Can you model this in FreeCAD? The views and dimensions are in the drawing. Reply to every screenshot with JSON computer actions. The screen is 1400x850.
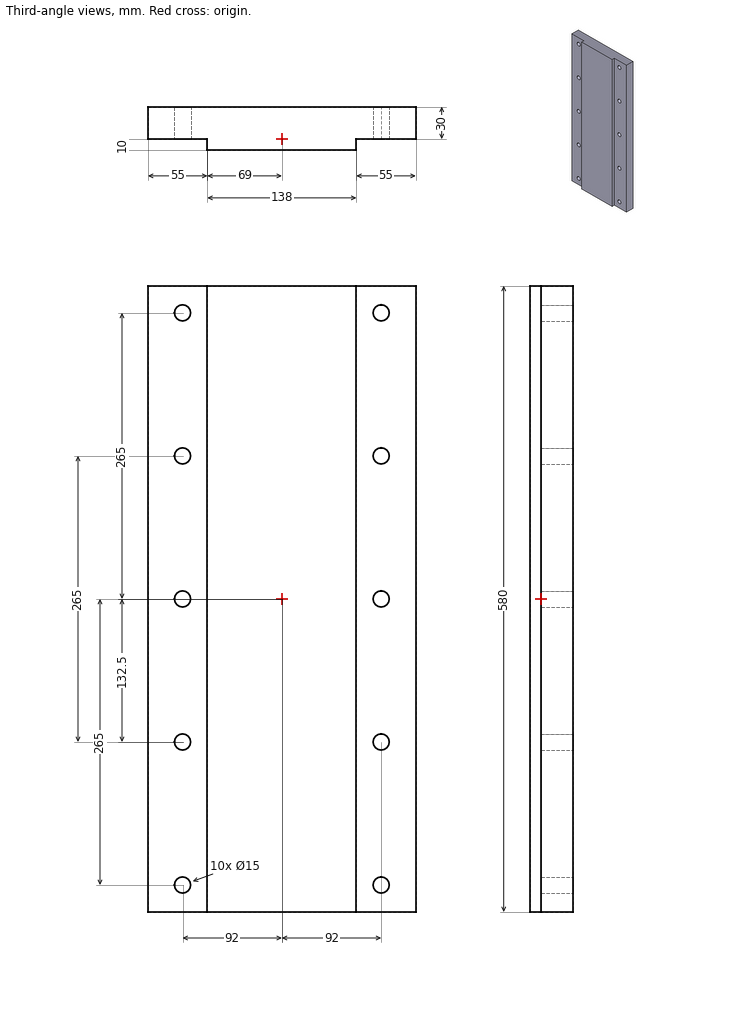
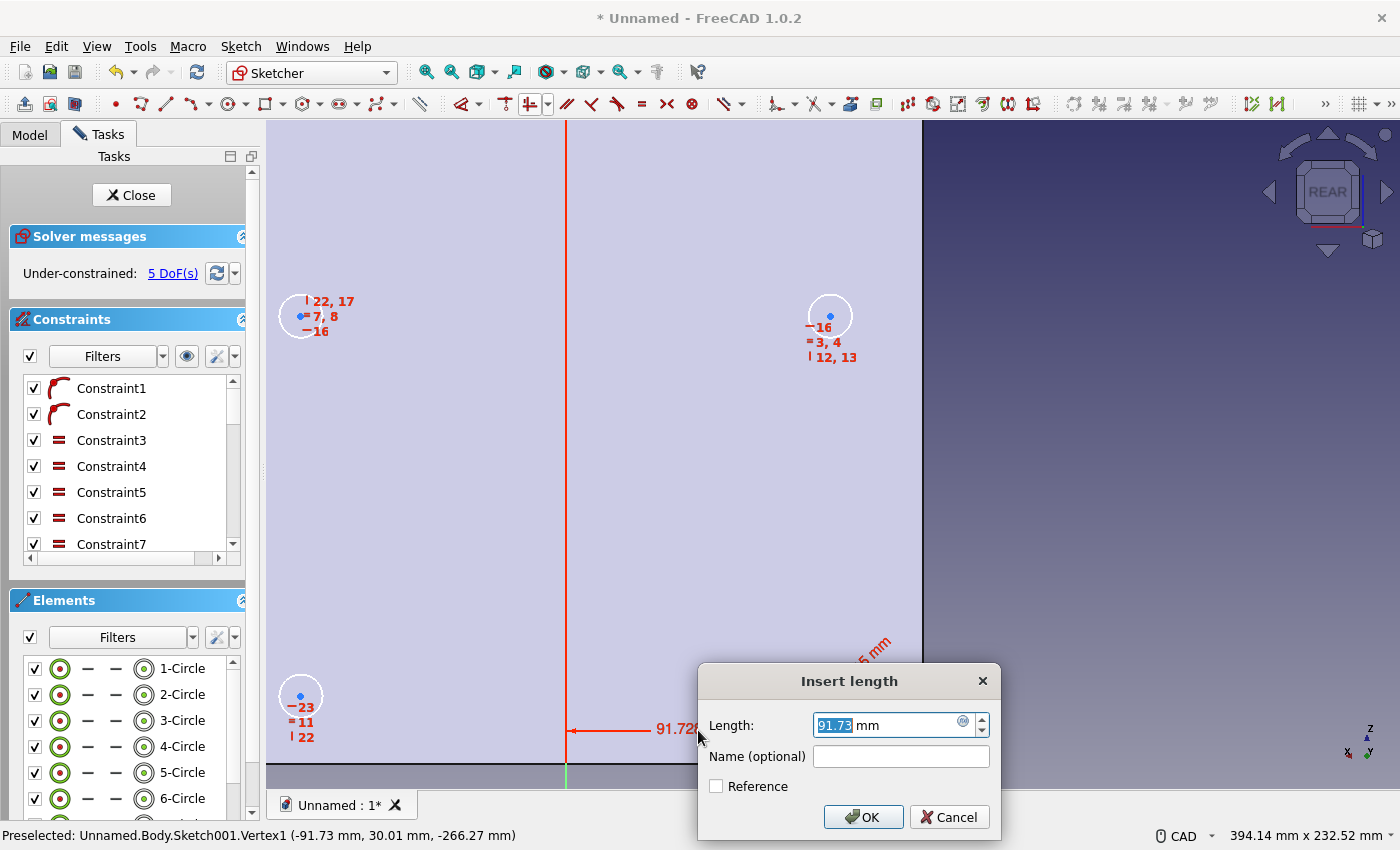
{"action": "type", "text": "92"}
{"action": "key", "text": "Return"}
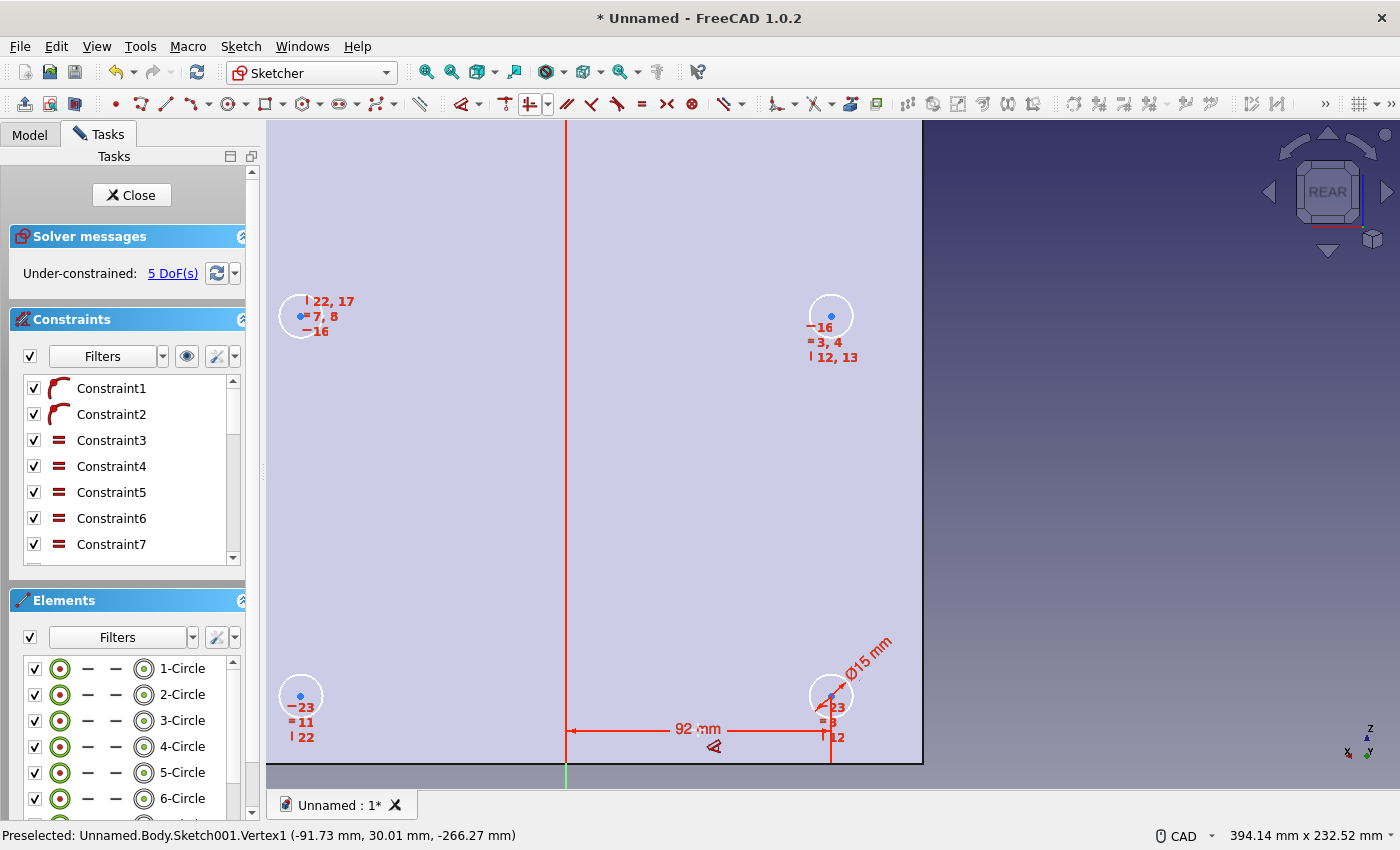
{"action": "left_click", "coordinate": [301, 316]}
{"action": "left_click", "coordinate": [434, 350]}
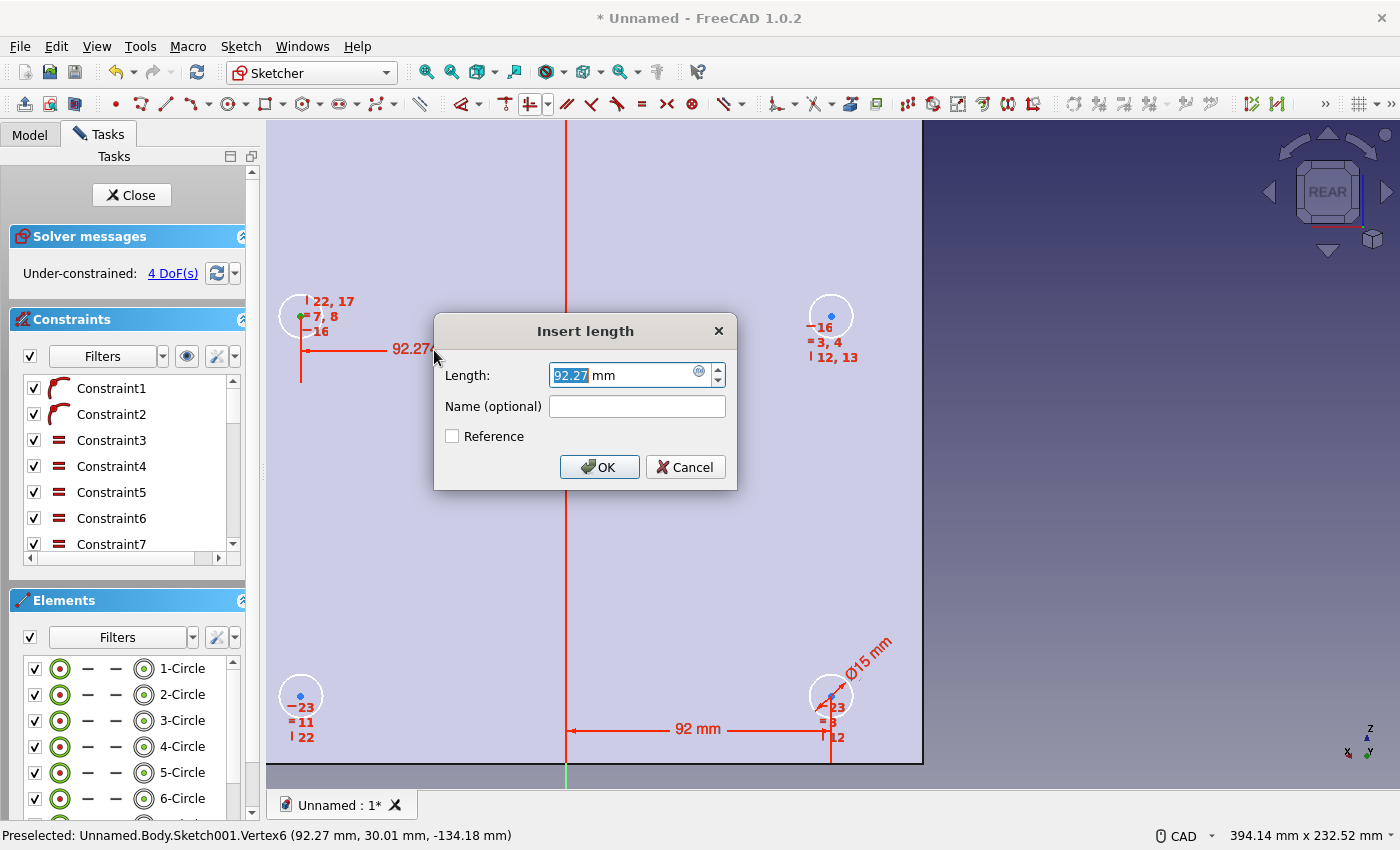
{"action": "type", "text": "92"}
{"action": "key", "text": "Return"}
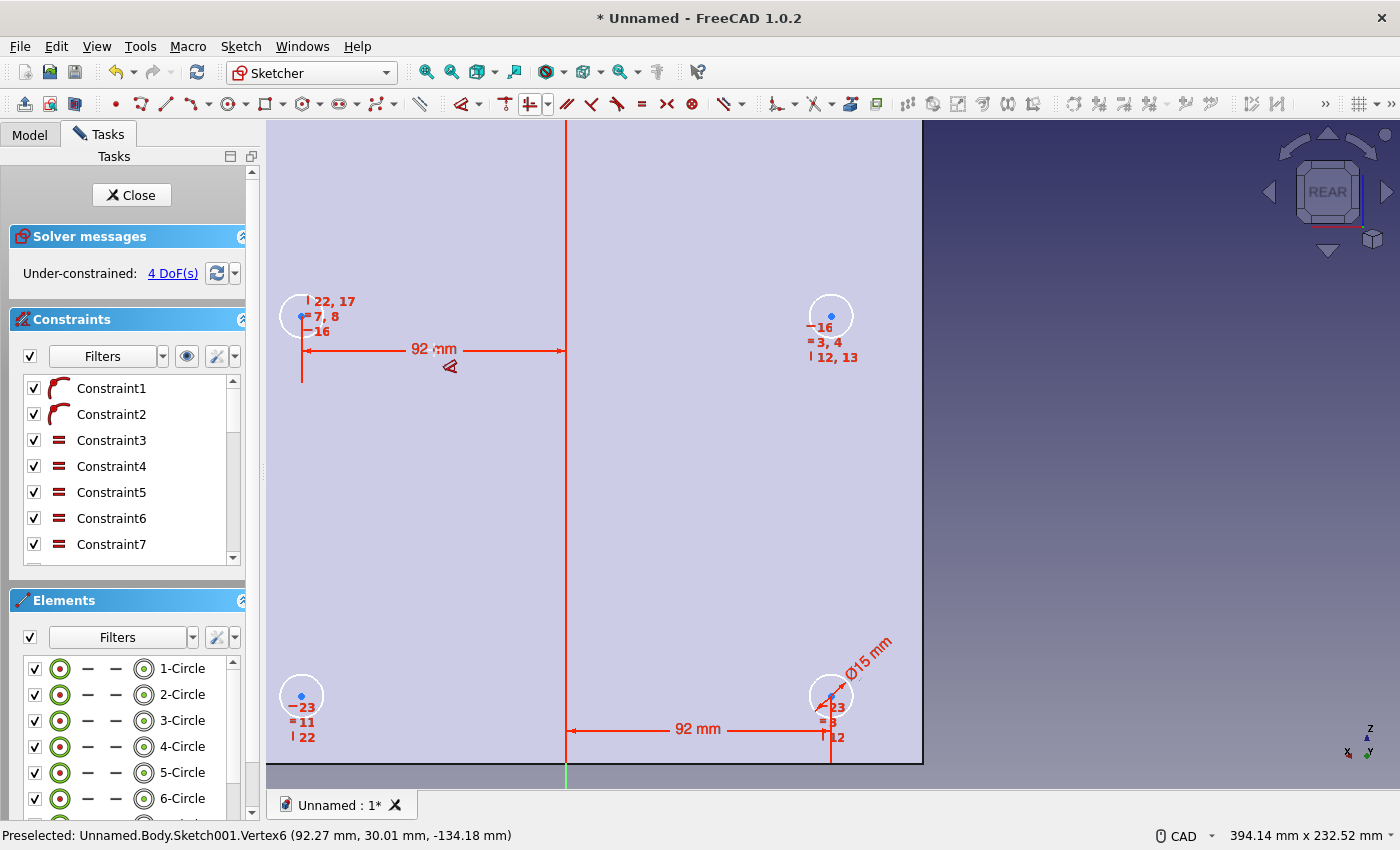
{"action": "left_click", "coordinate": [831, 696]}
{"action": "left_click", "coordinate": [865, 422]}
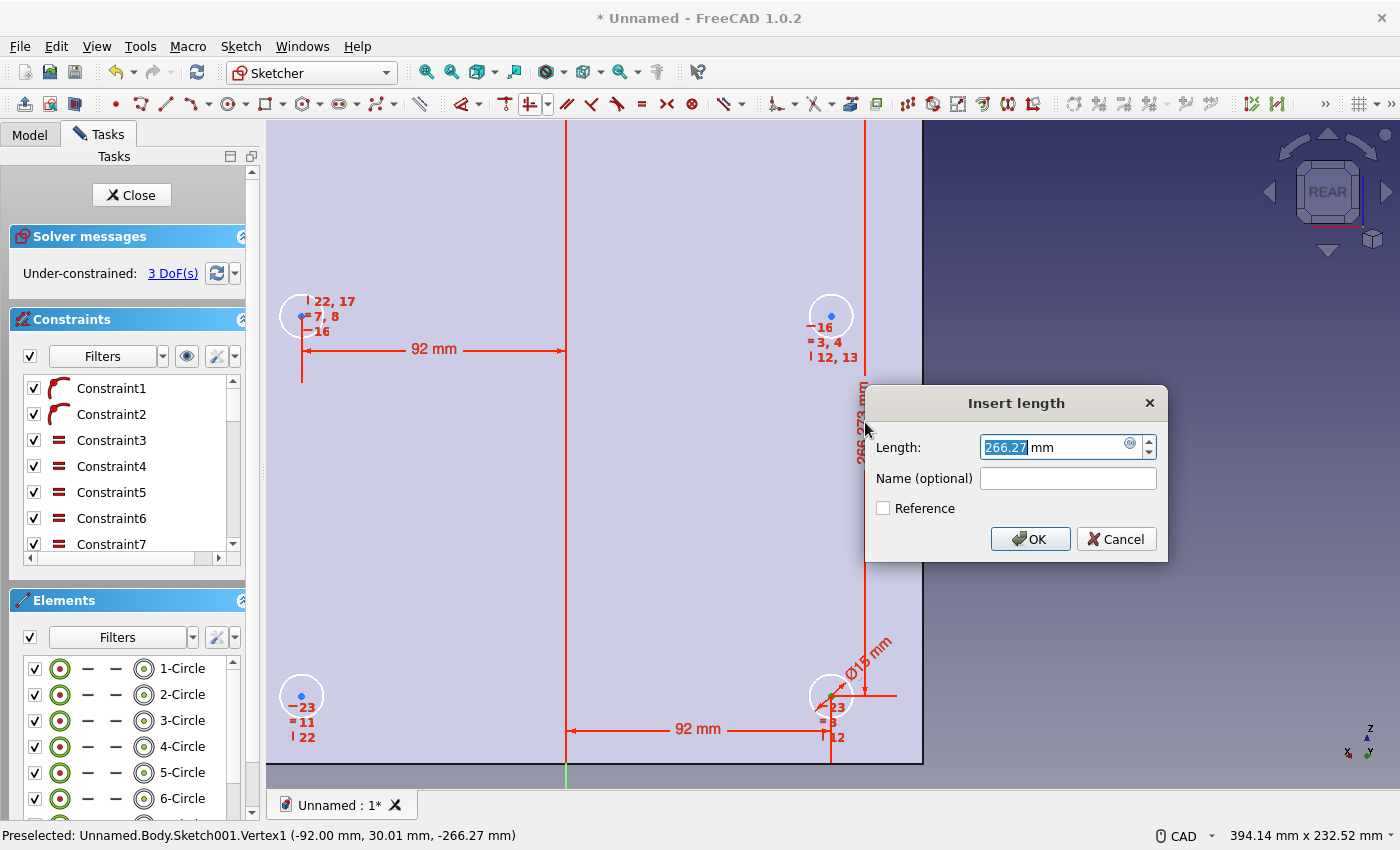
{"action": "type", "text": "265"}
{"action": "key", "text": "Return"}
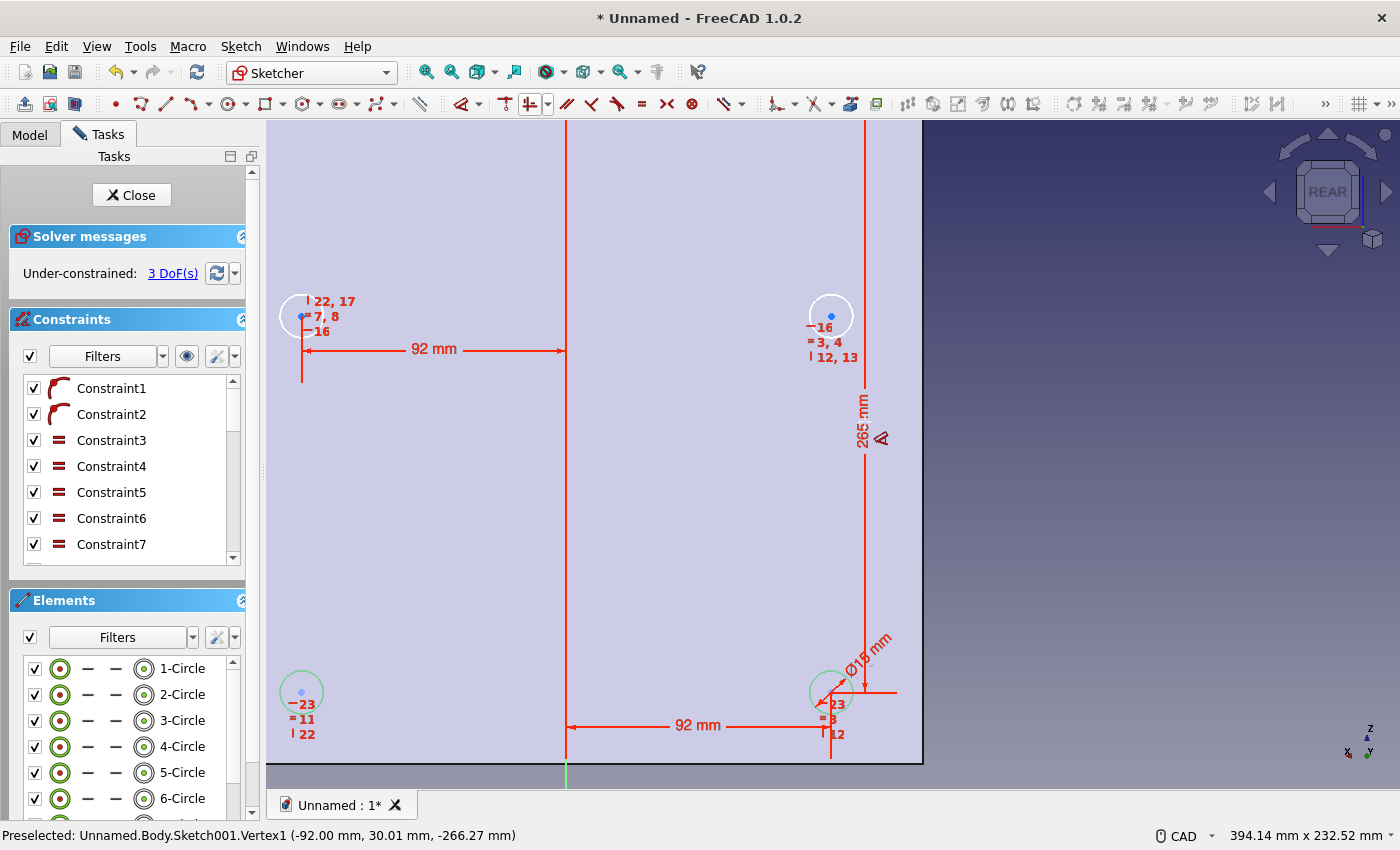
{"action": "scroll", "coordinate": [850, 681], "scroll_direction": "down", "scroll_amount": 6}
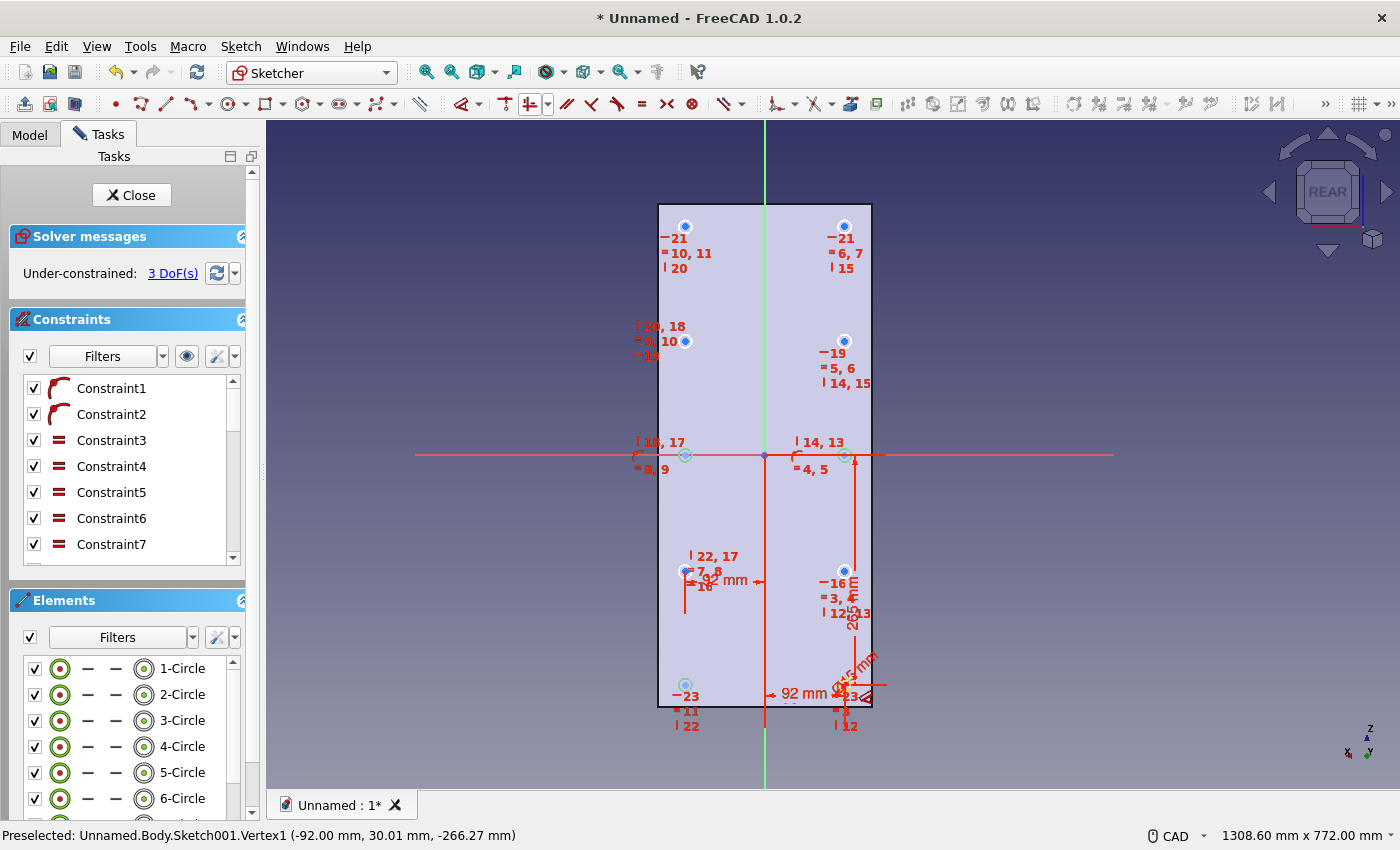
{"action": "left_click", "coordinate": [845, 227]}
{"action": "left_click", "coordinate": [879, 341]}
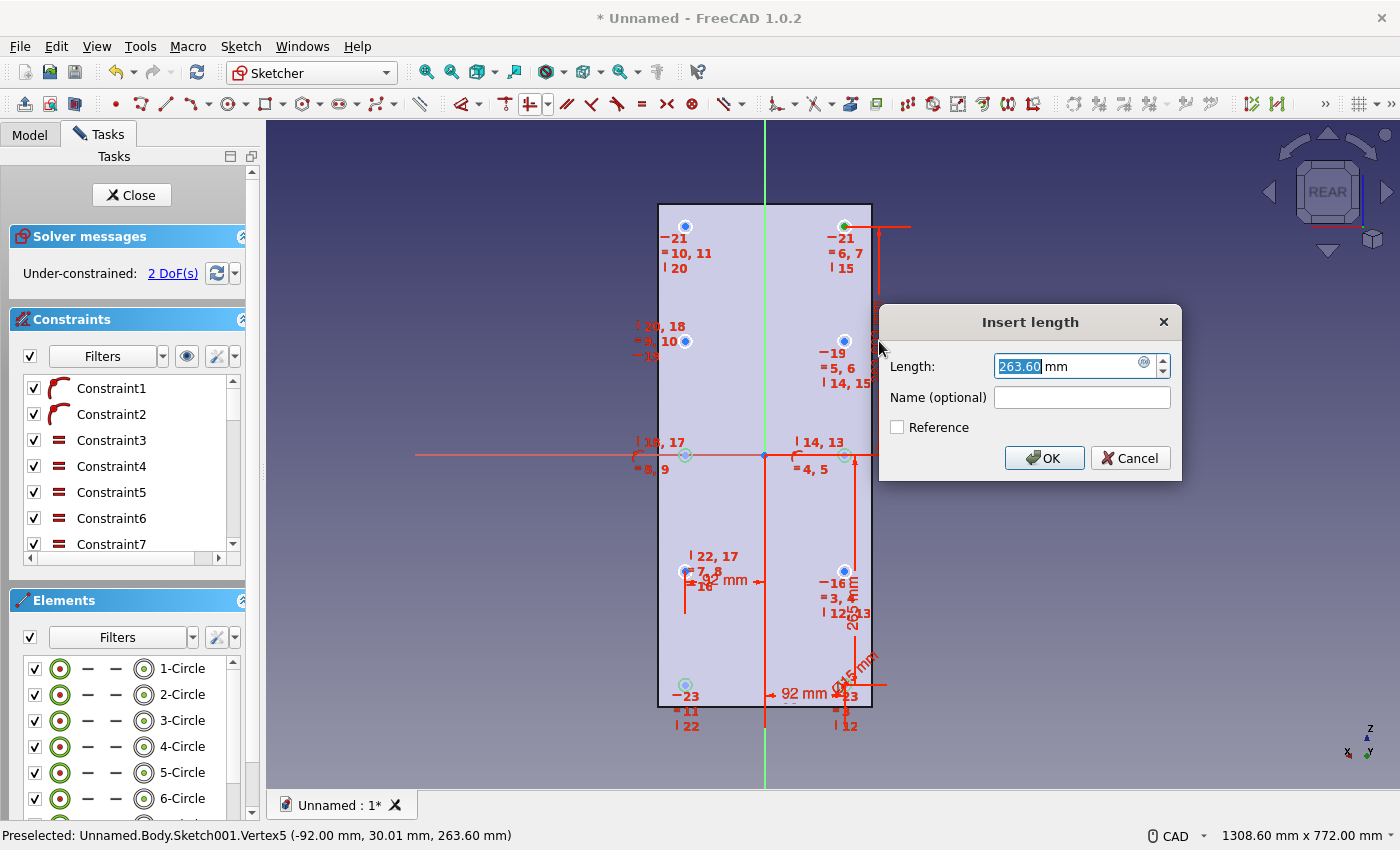
{"action": "type", "text": "265"}
{"action": "key", "text": "Return"}